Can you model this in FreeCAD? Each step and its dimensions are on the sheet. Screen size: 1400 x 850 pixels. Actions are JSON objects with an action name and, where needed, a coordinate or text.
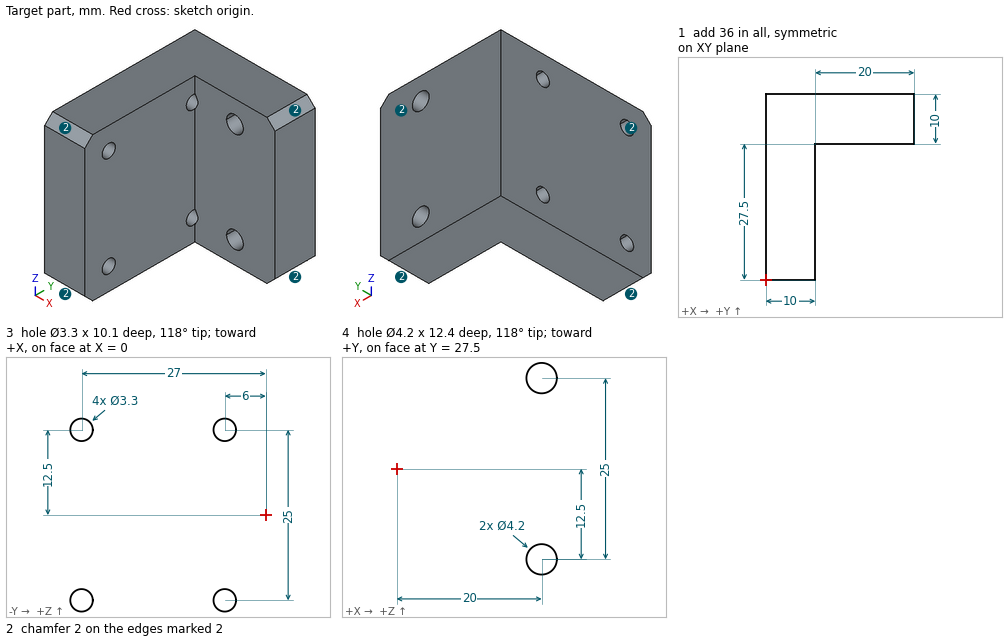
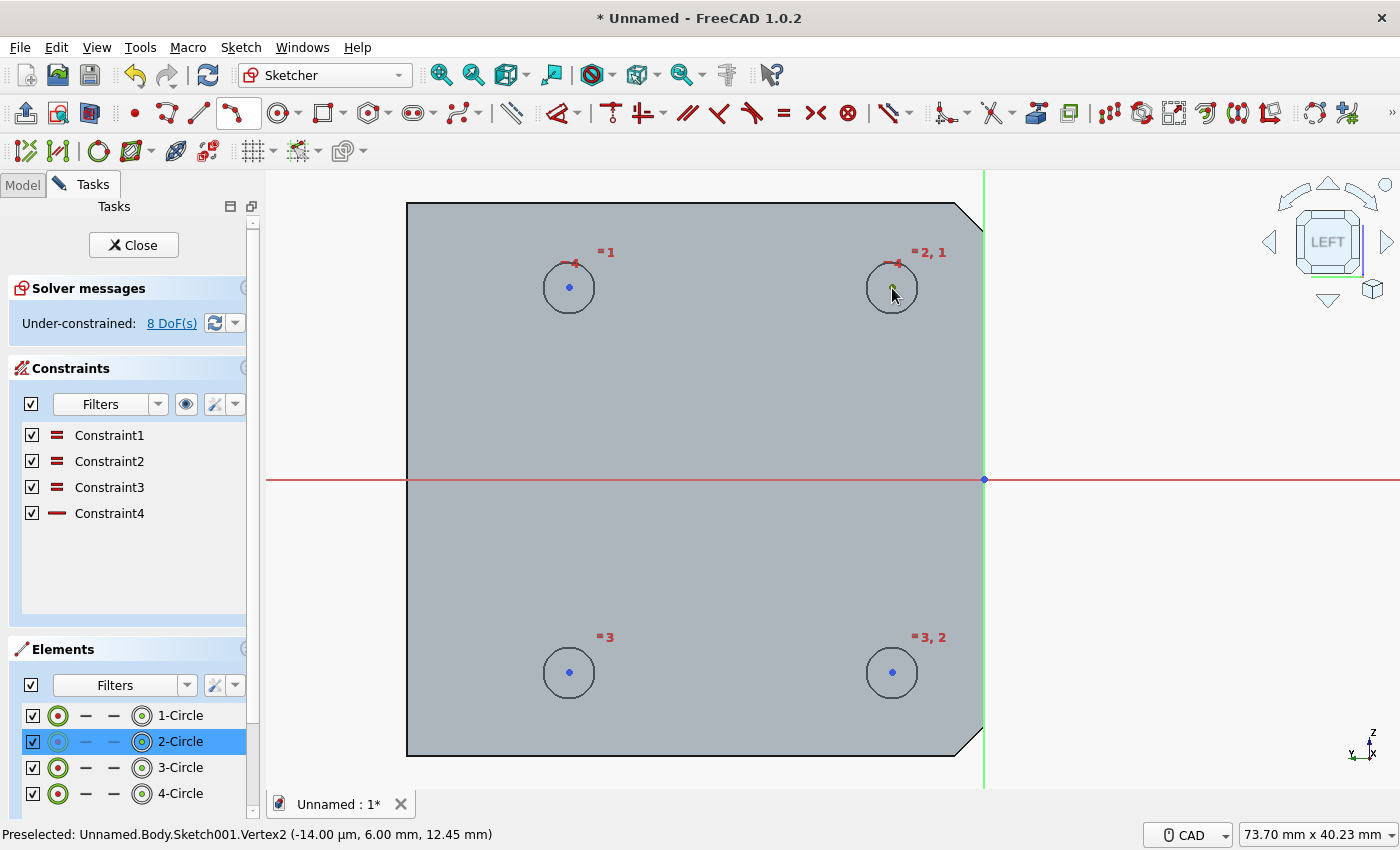
{"action": "left_click", "coordinate": [892, 673]}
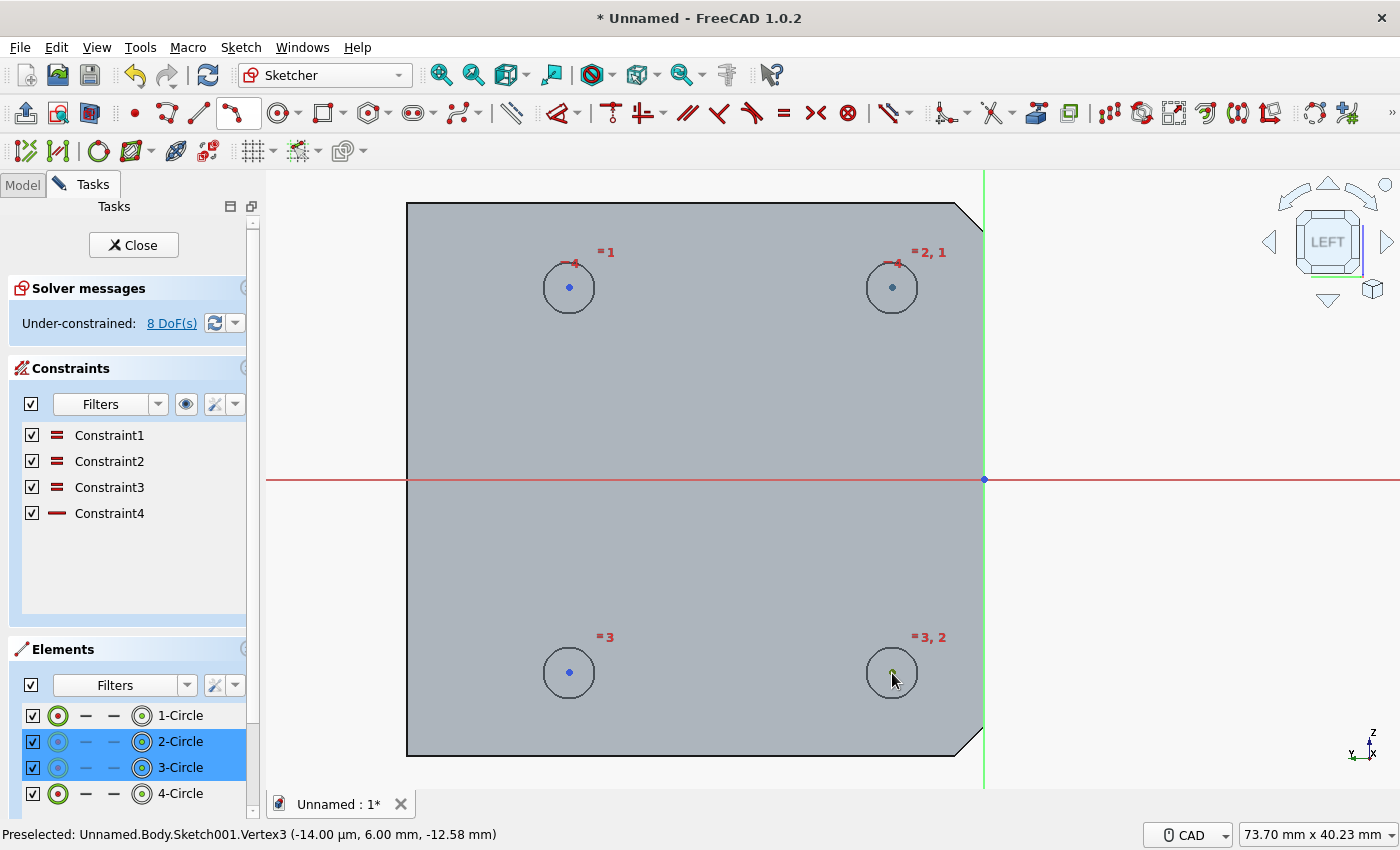
{"action": "key", "text": "v"}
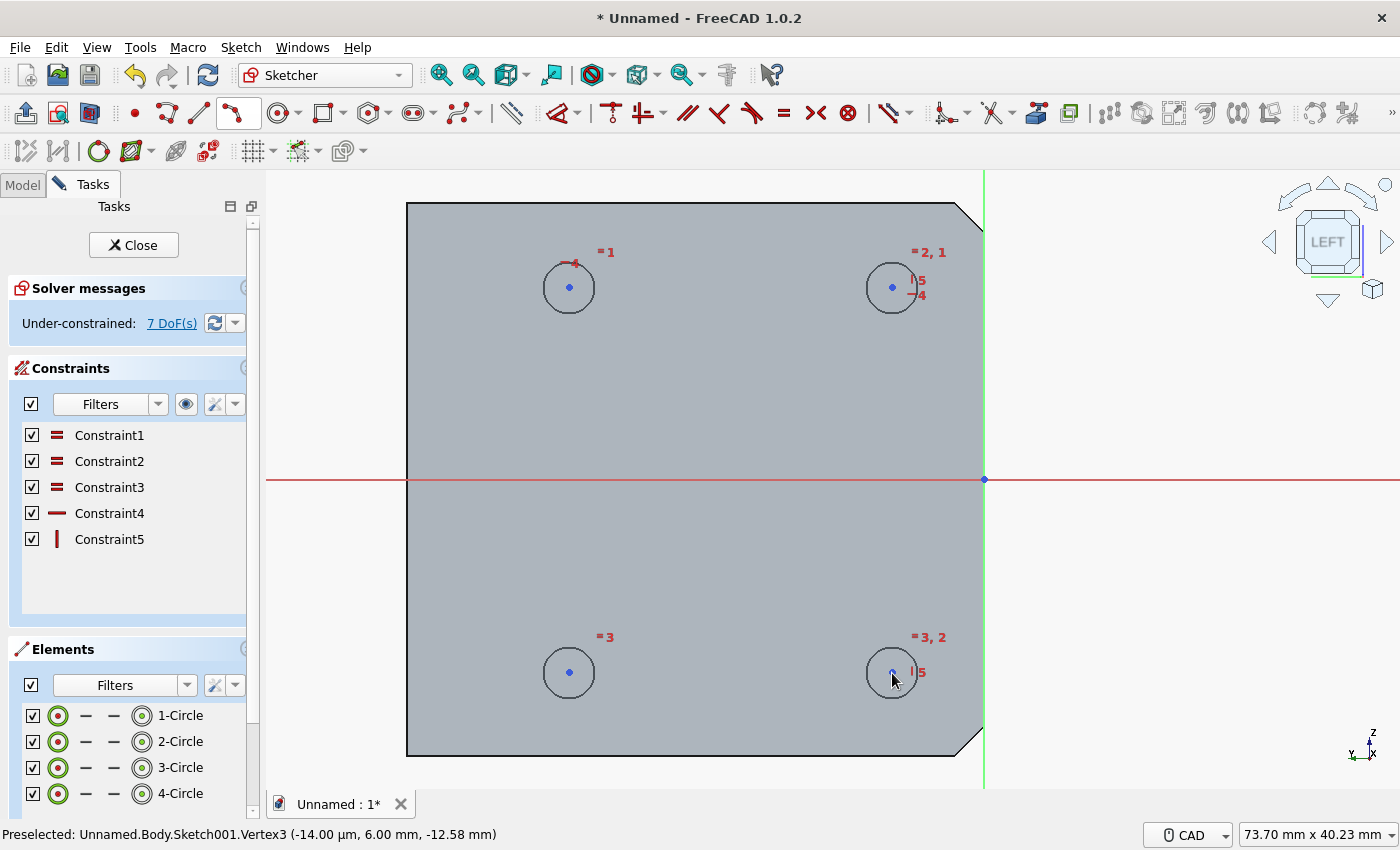
{"action": "left_click", "coordinate": [569, 288]}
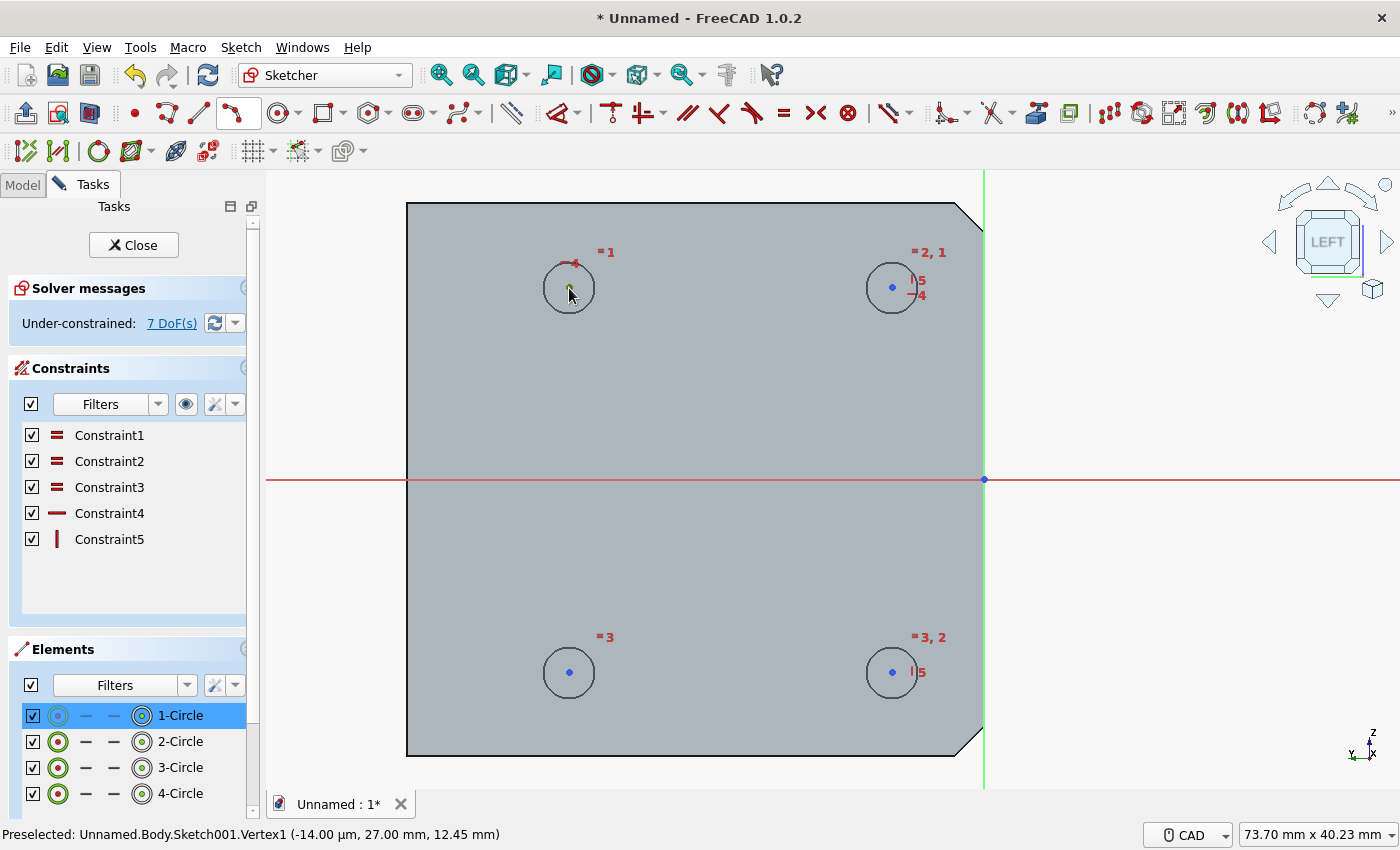
{"action": "left_click", "coordinate": [569, 673]}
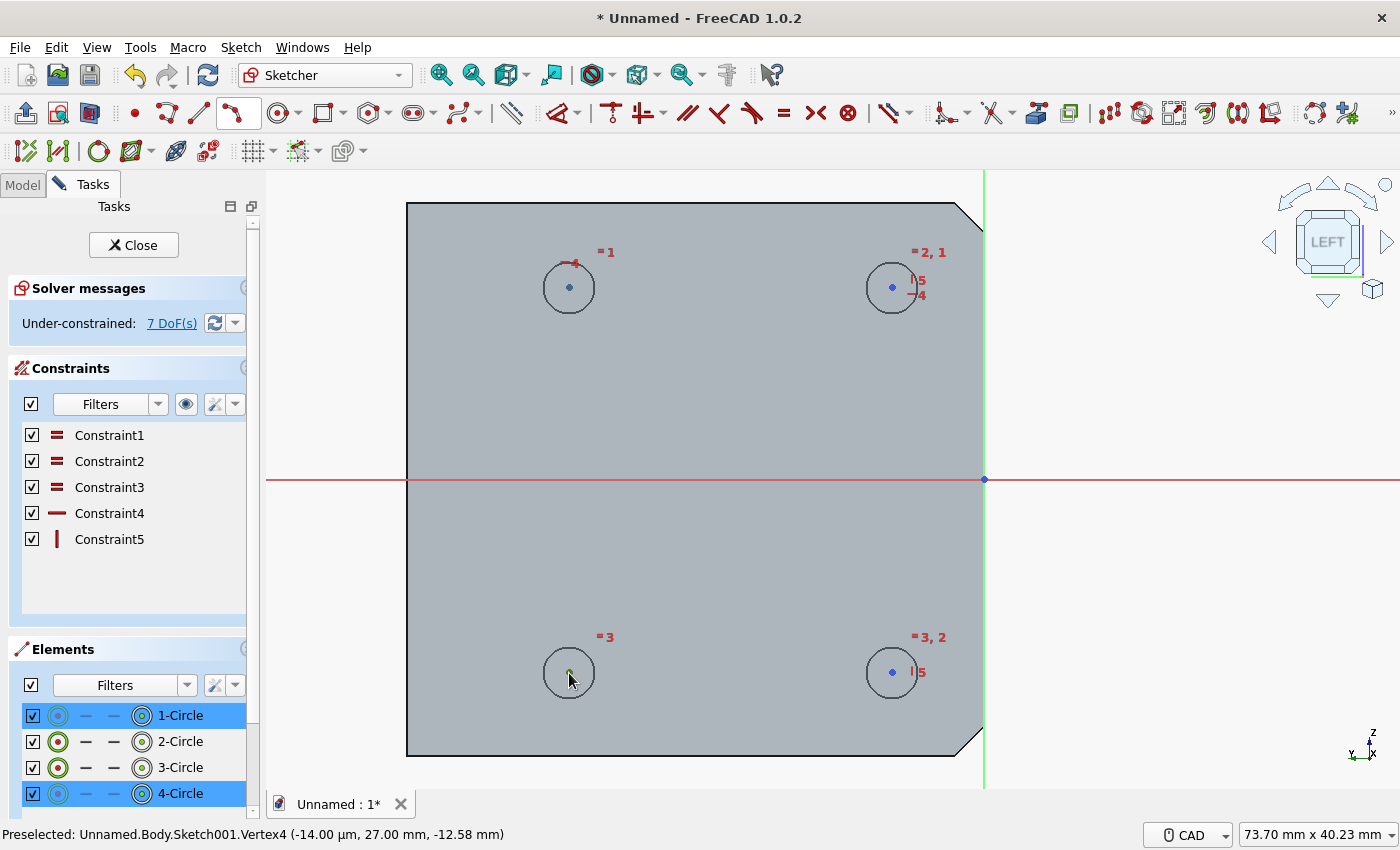
{"action": "key", "text": "v"}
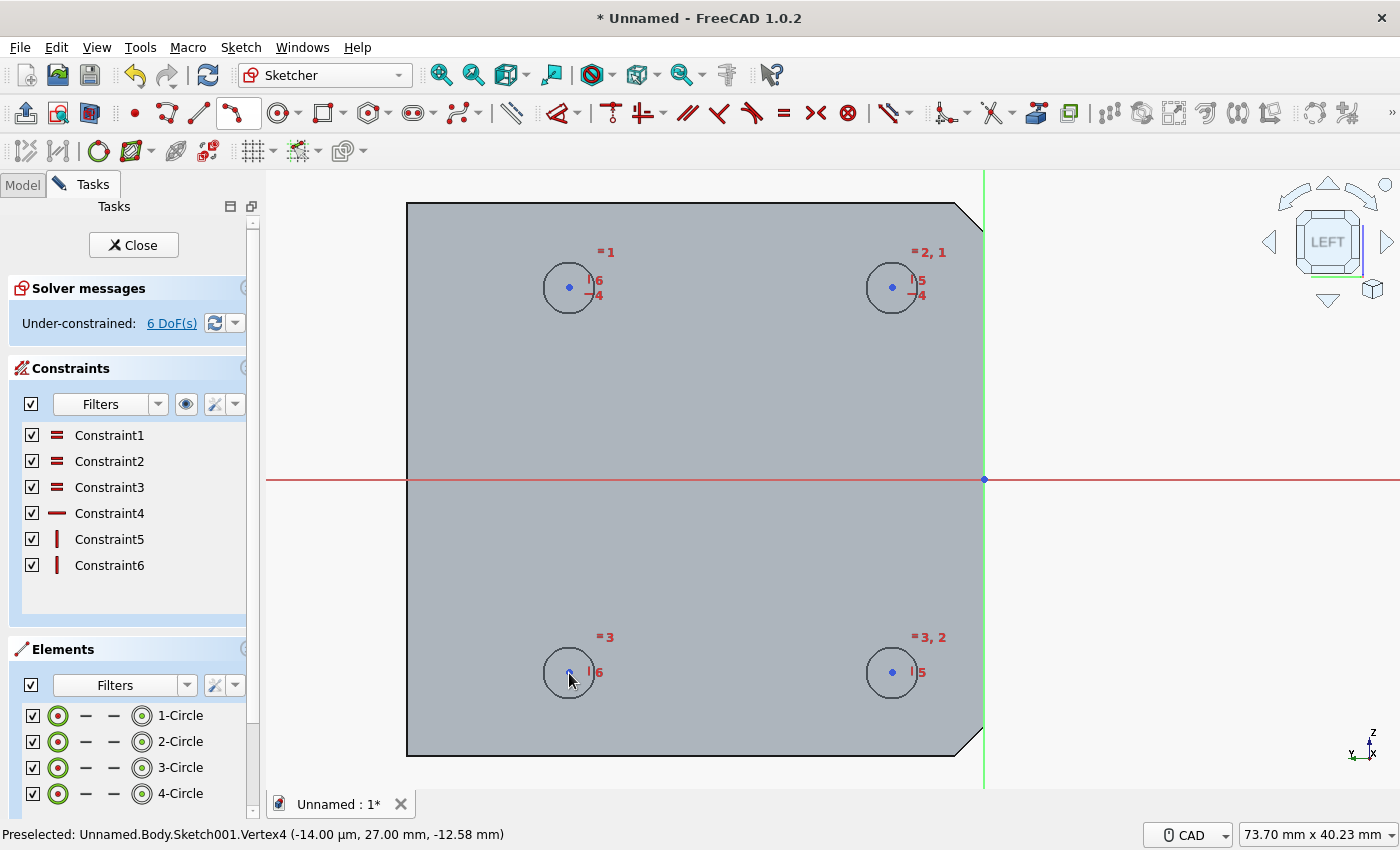
{"action": "left_click", "coordinate": [892, 673]}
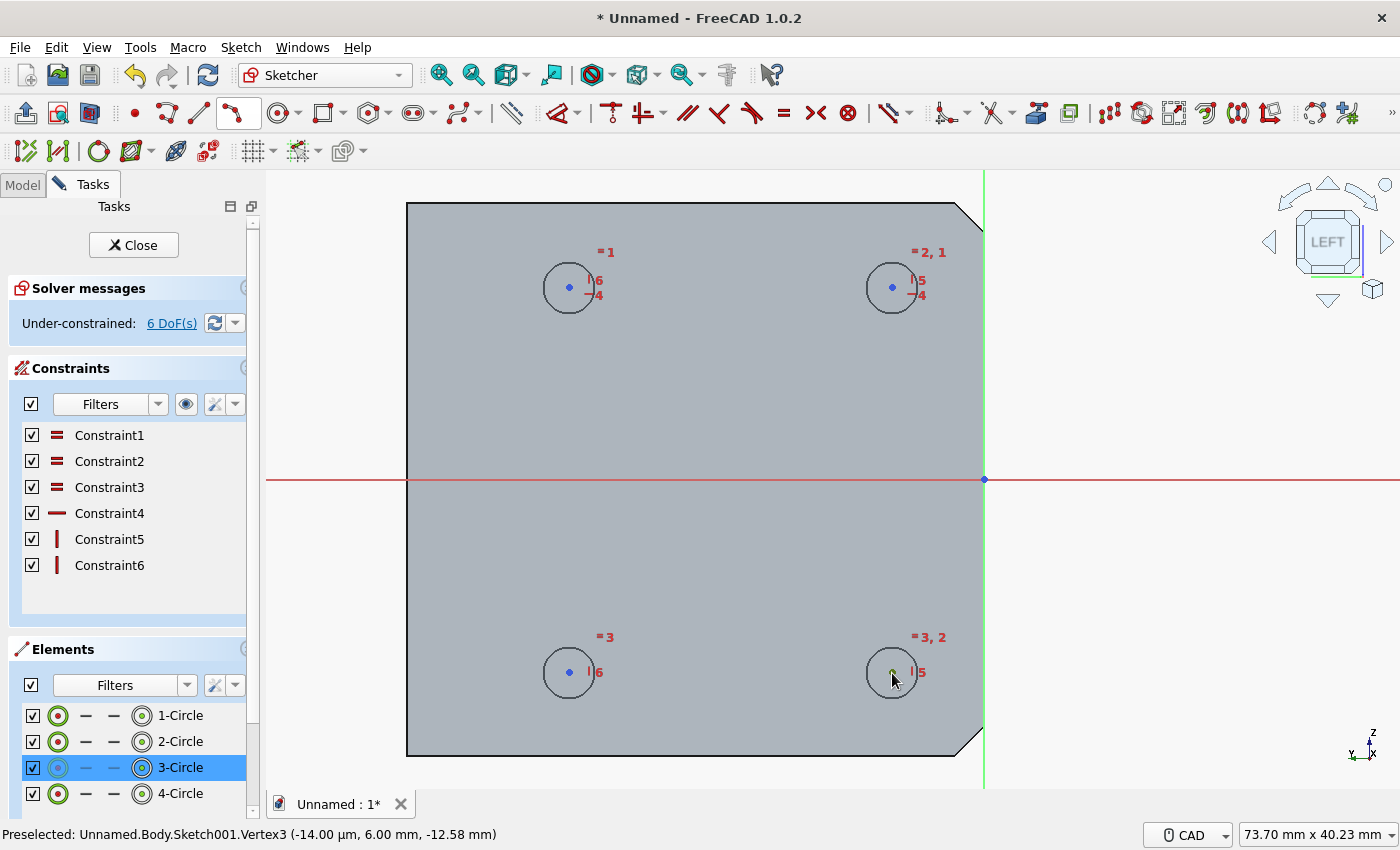
{"action": "left_click", "coordinate": [569, 673]}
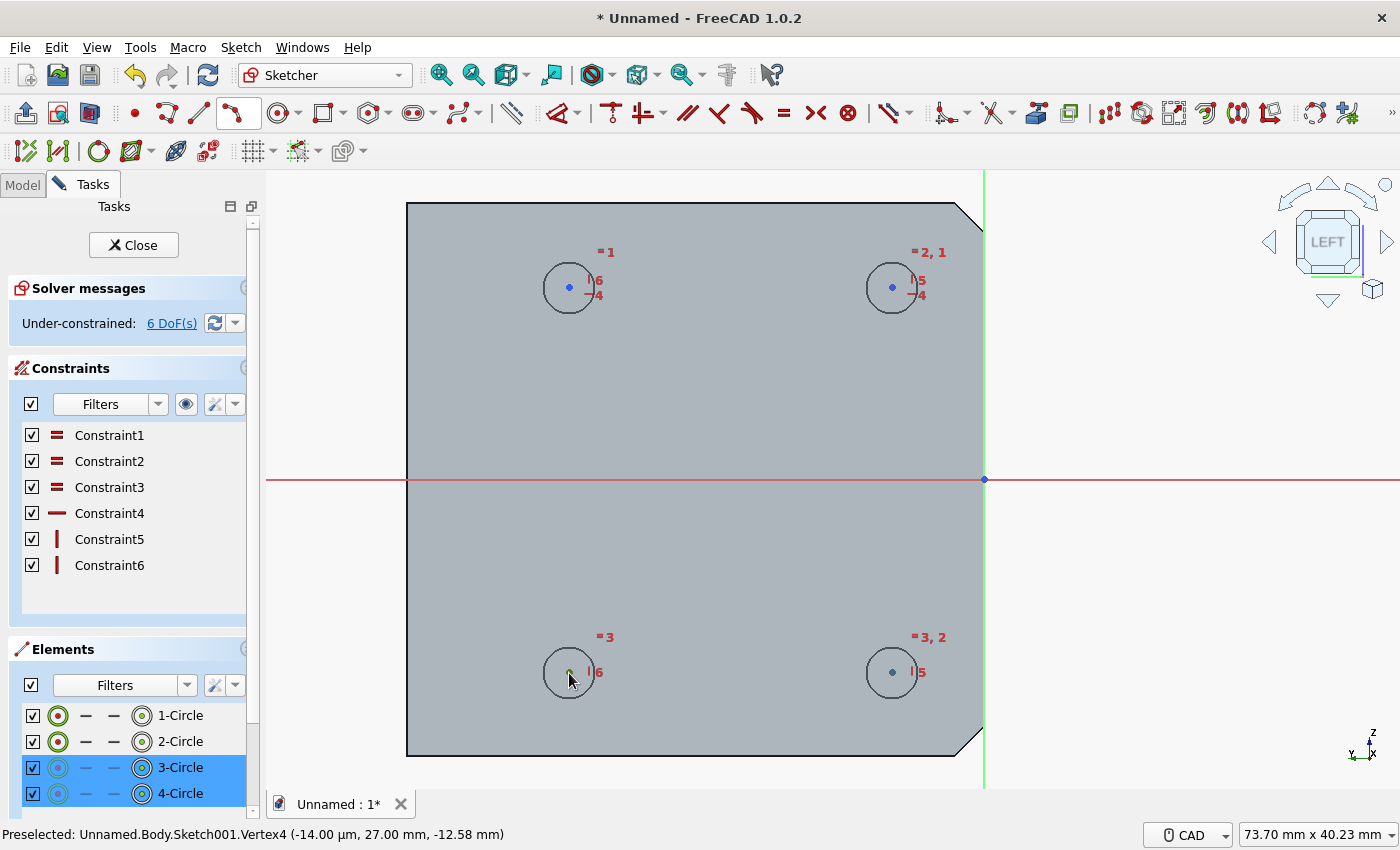
{"action": "left_click", "coordinate": [666, 114]}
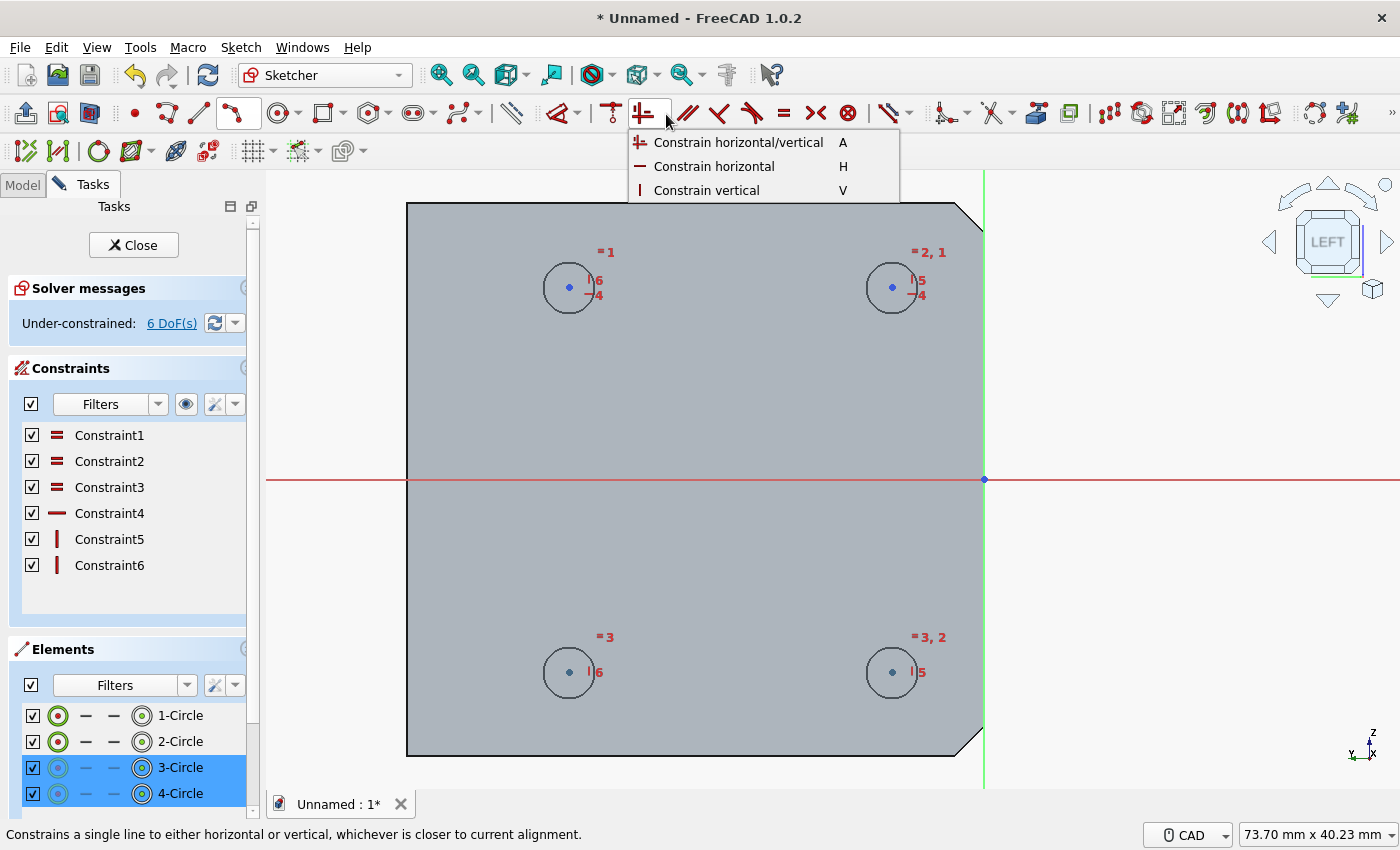
{"action": "left_click", "coordinate": [764, 166]}